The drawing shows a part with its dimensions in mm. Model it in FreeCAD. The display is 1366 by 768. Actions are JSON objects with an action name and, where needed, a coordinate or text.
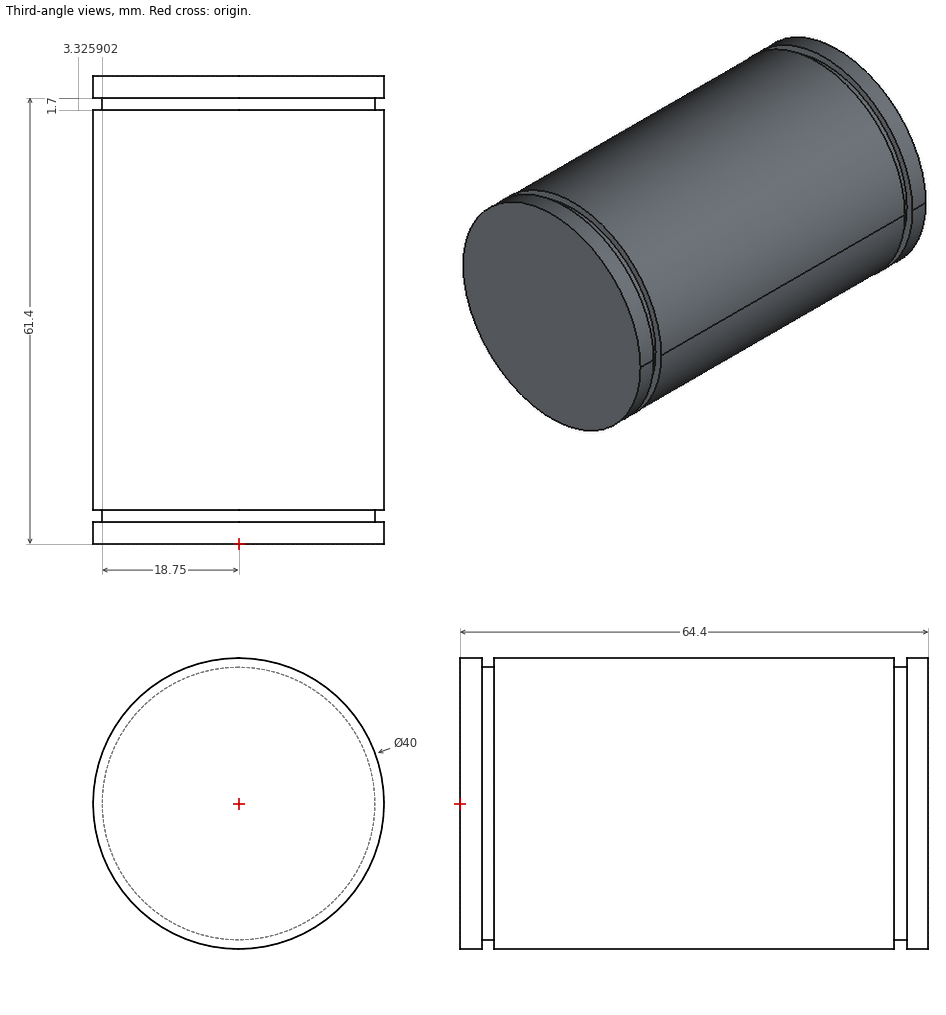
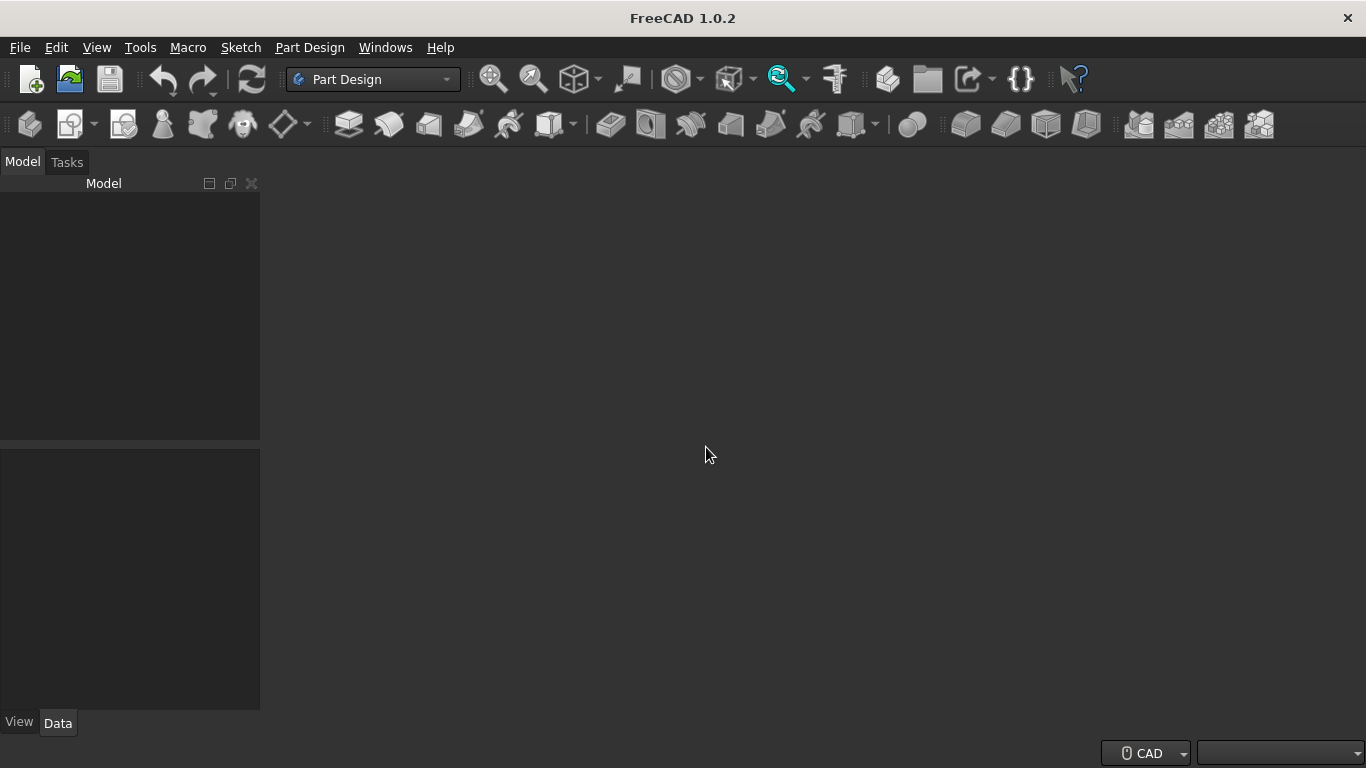
{"action": "left_click", "coordinate": [30, 80]}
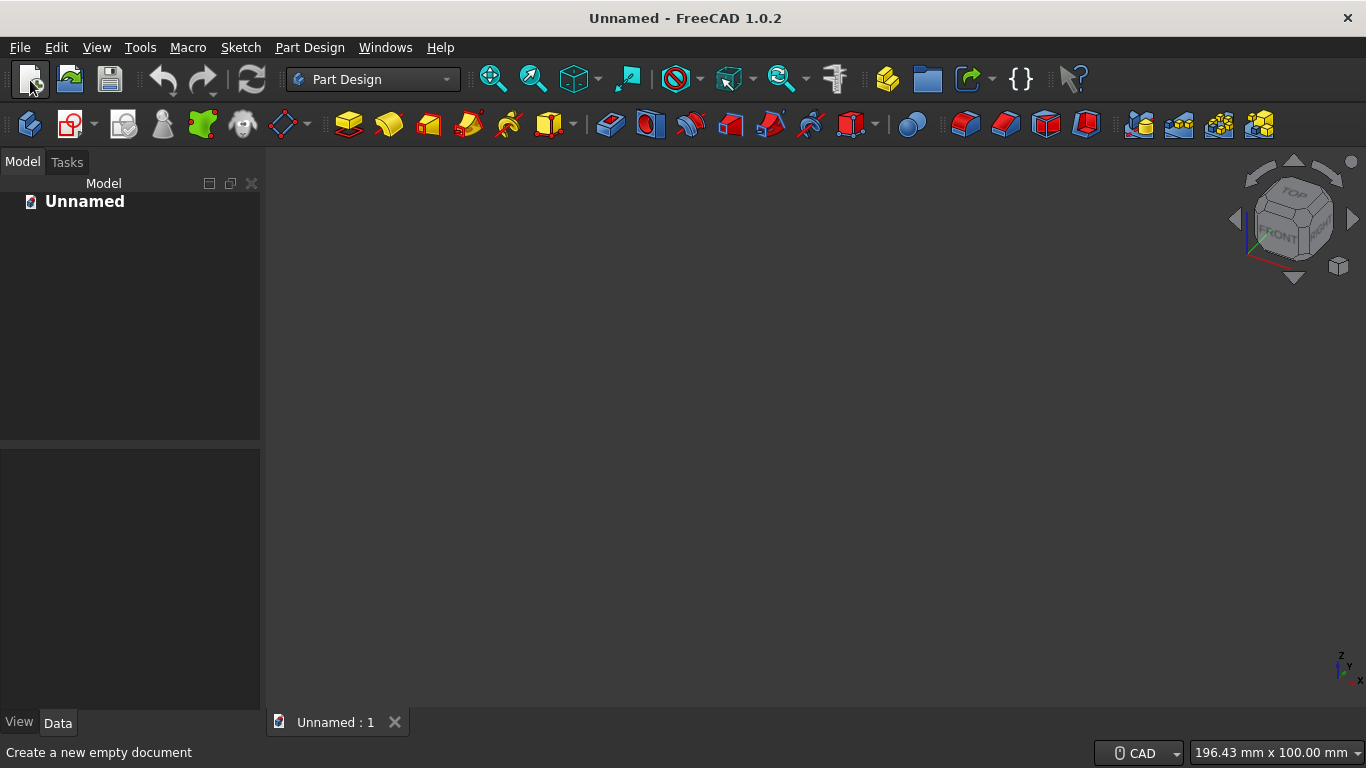
{"action": "left_click", "coordinate": [70, 124]}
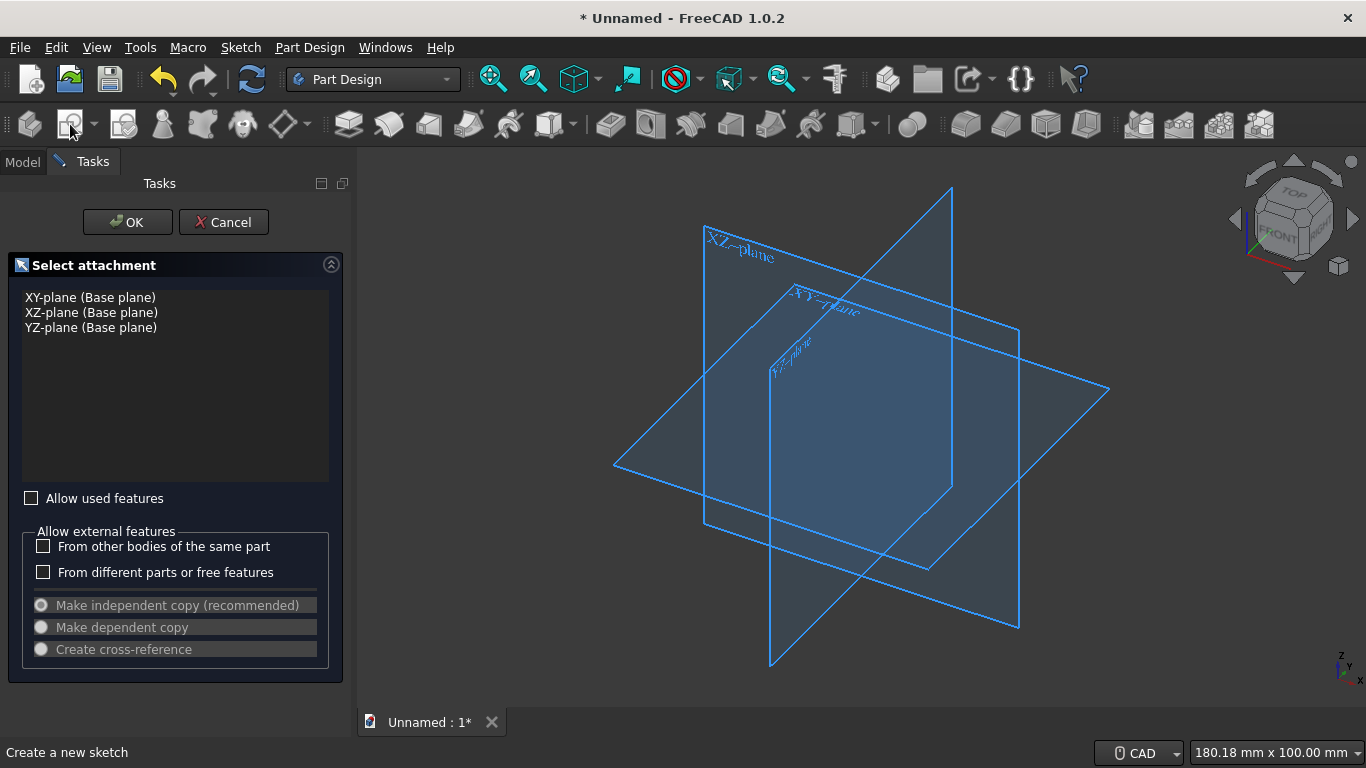
{"action": "left_click", "coordinate": [82, 312]}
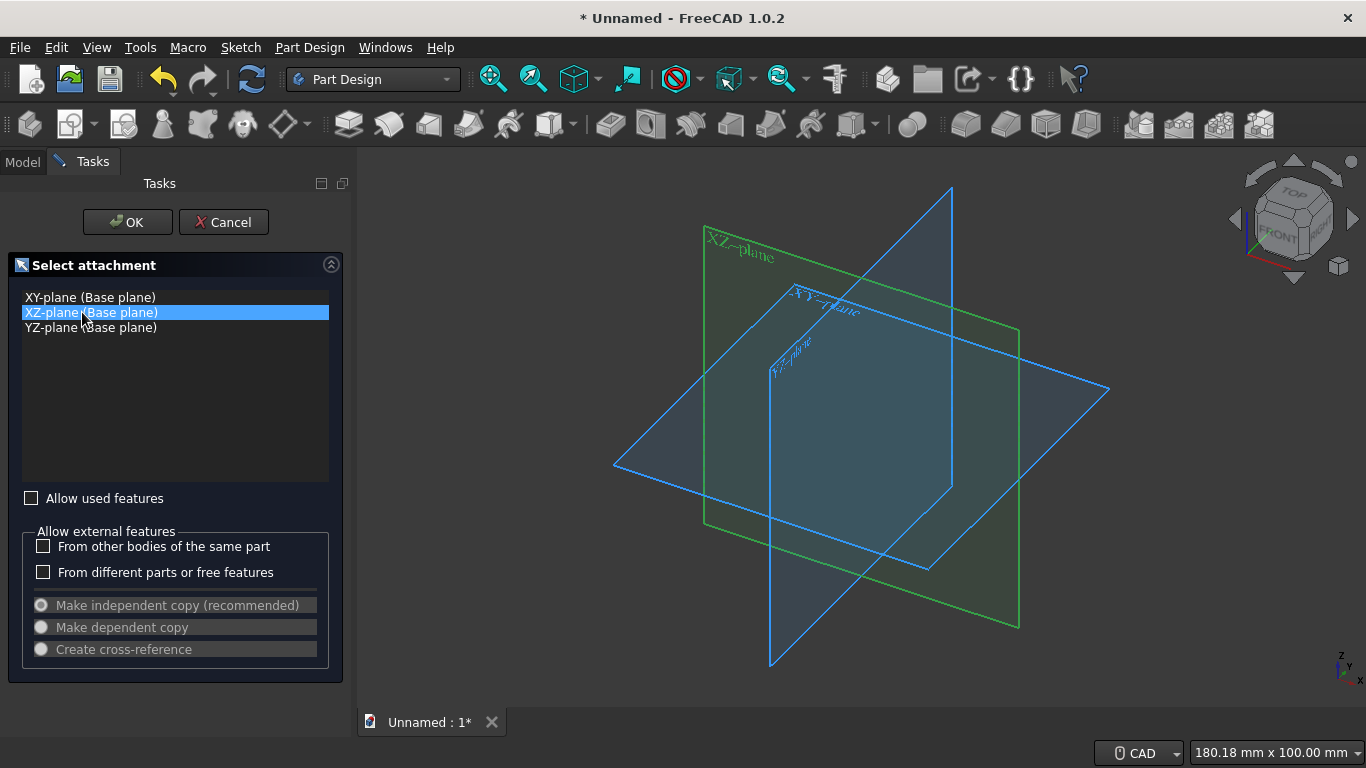
{"action": "left_click", "coordinate": [128, 222]}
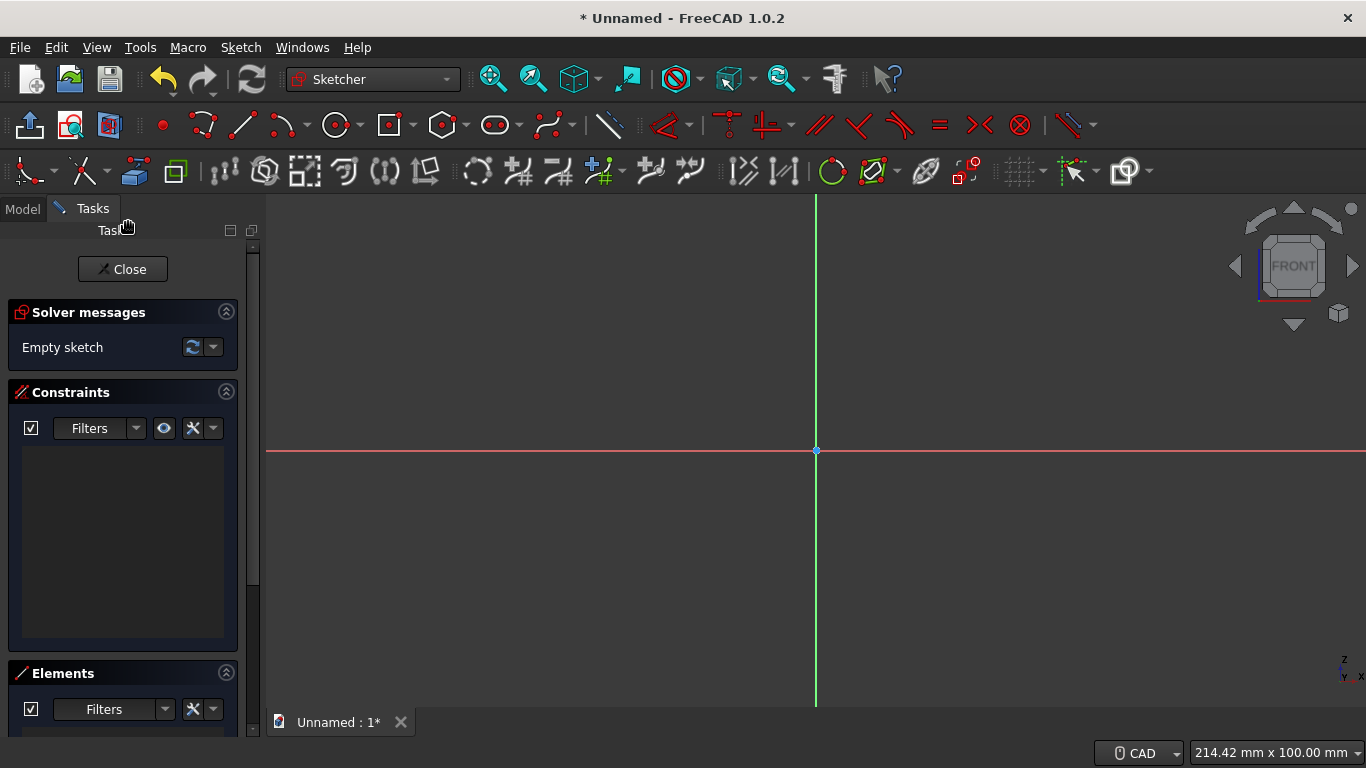
{"action": "scroll", "coordinate": [955, 451], "scroll_direction": "up", "scroll_amount": 2}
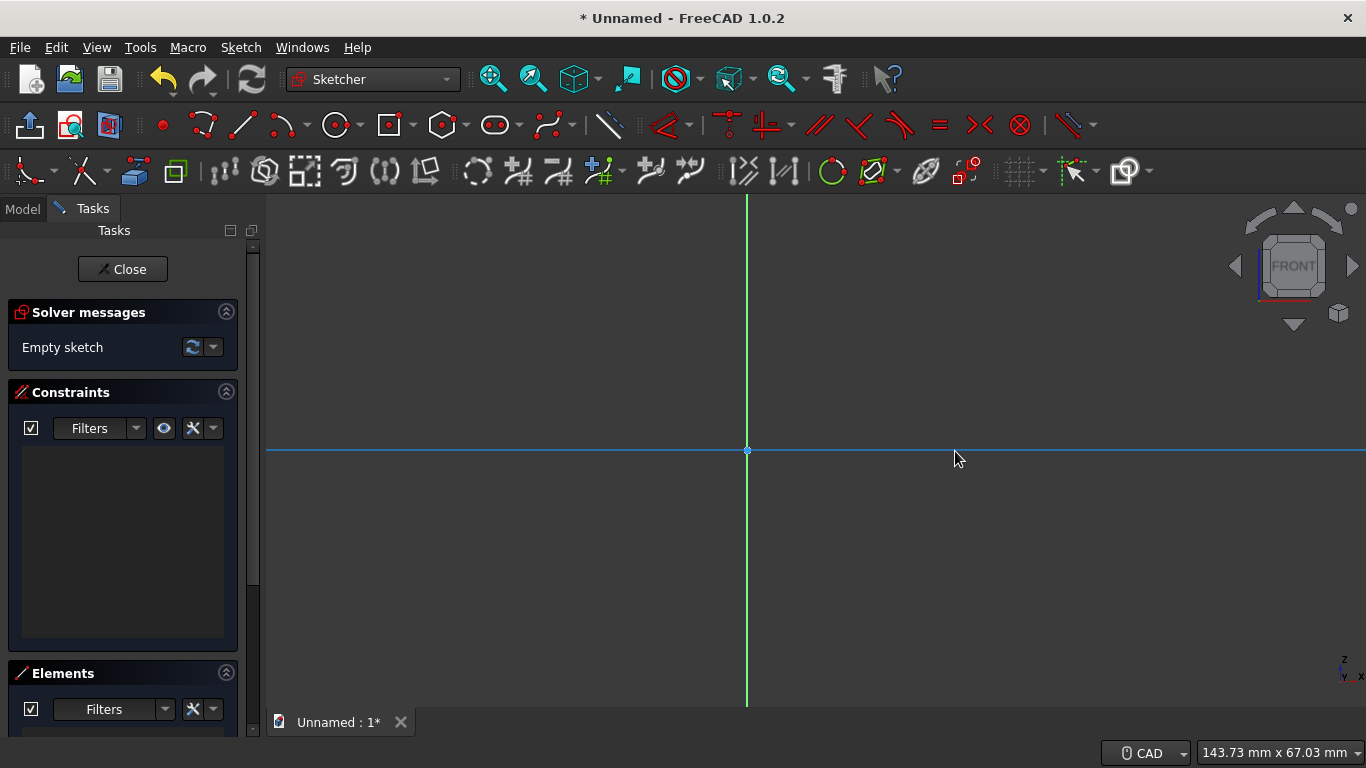
{"action": "left_click", "coordinate": [336, 126]}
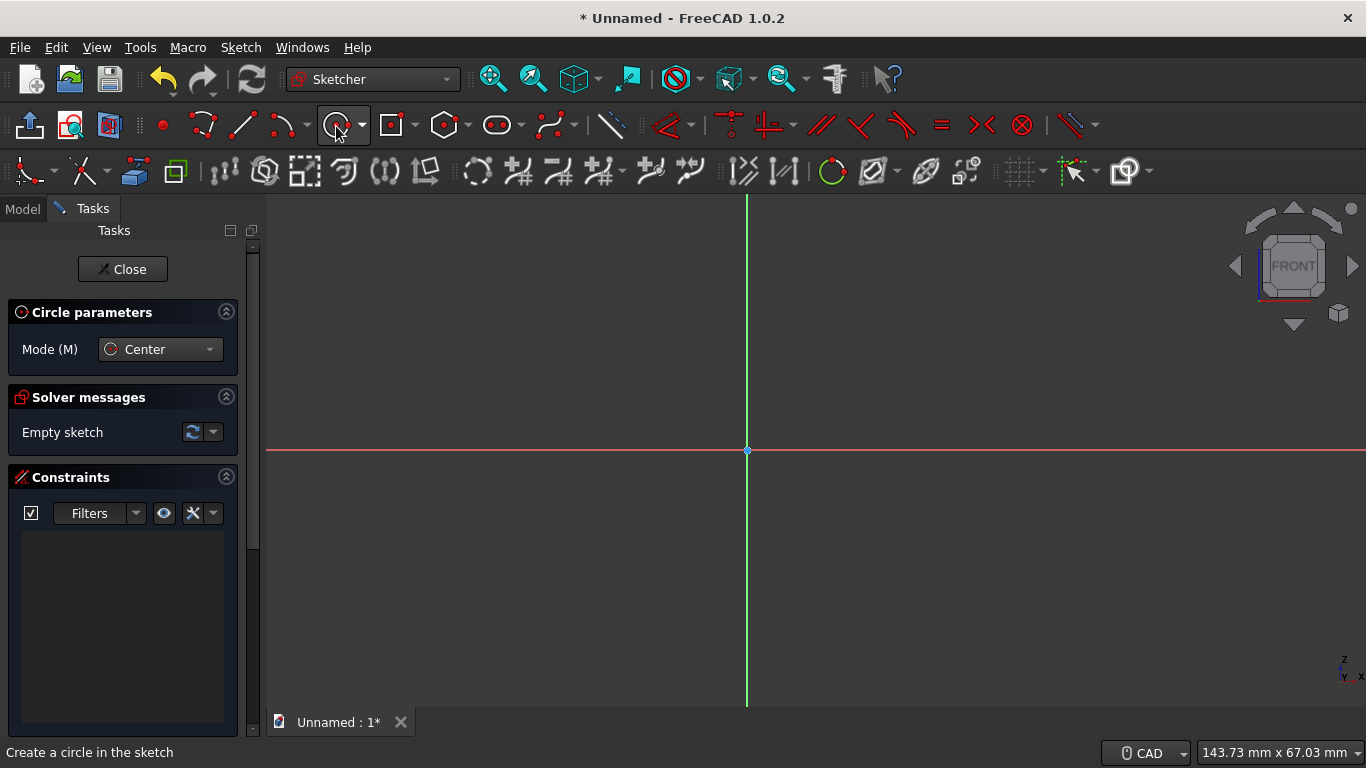
{"action": "left_click", "coordinate": [747, 450]}
{"action": "mouse_move", "coordinate": [856, 342]}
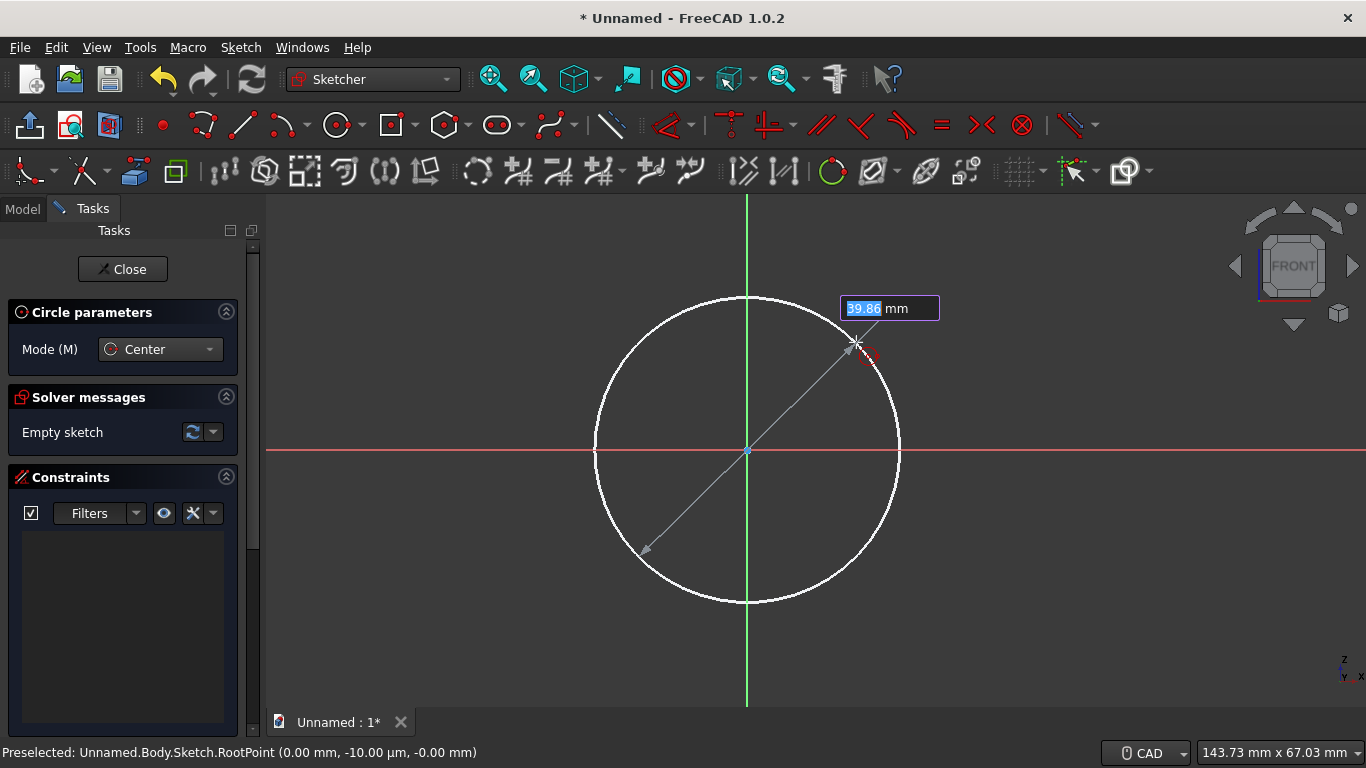
{"action": "type", "text": "40"}
{"action": "key", "text": "Return"}
{"action": "key", "text": "Escape"}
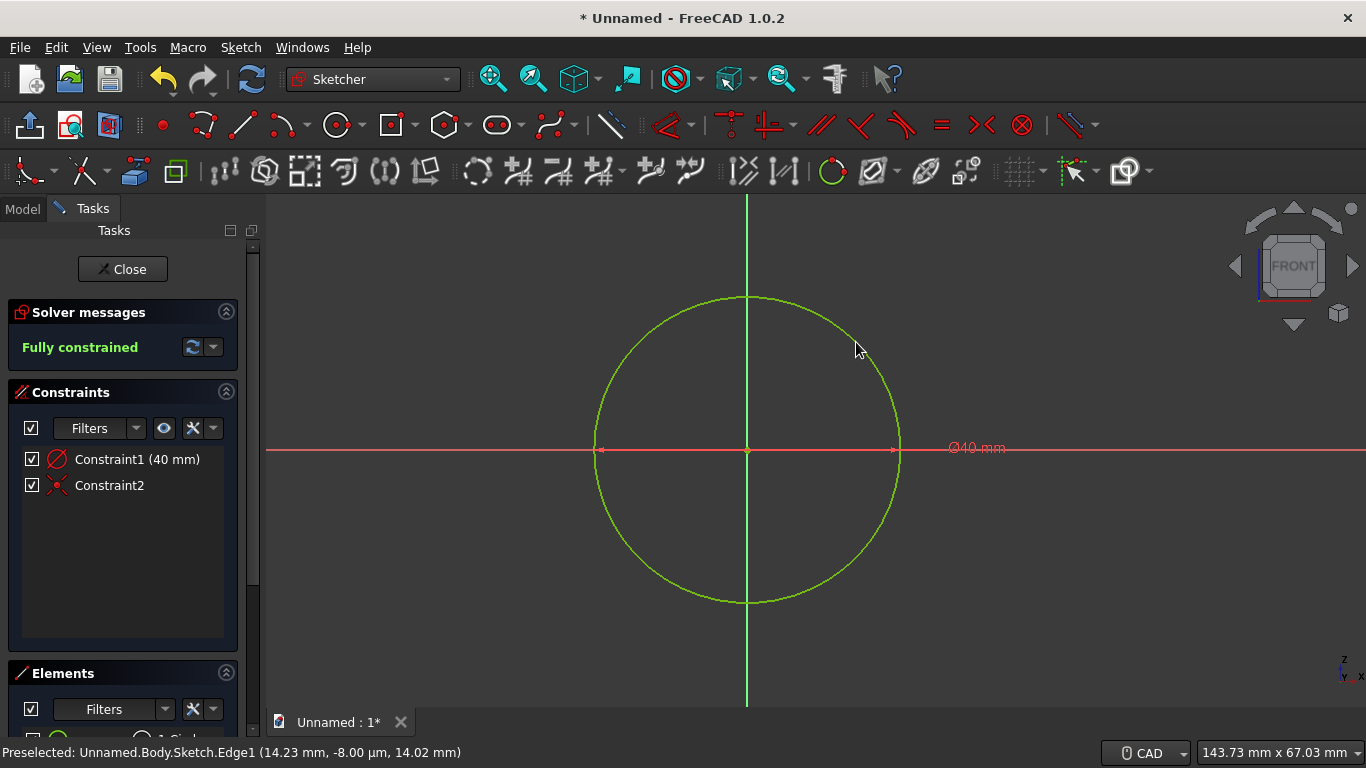
{"action": "left_click", "coordinate": [123, 269]}